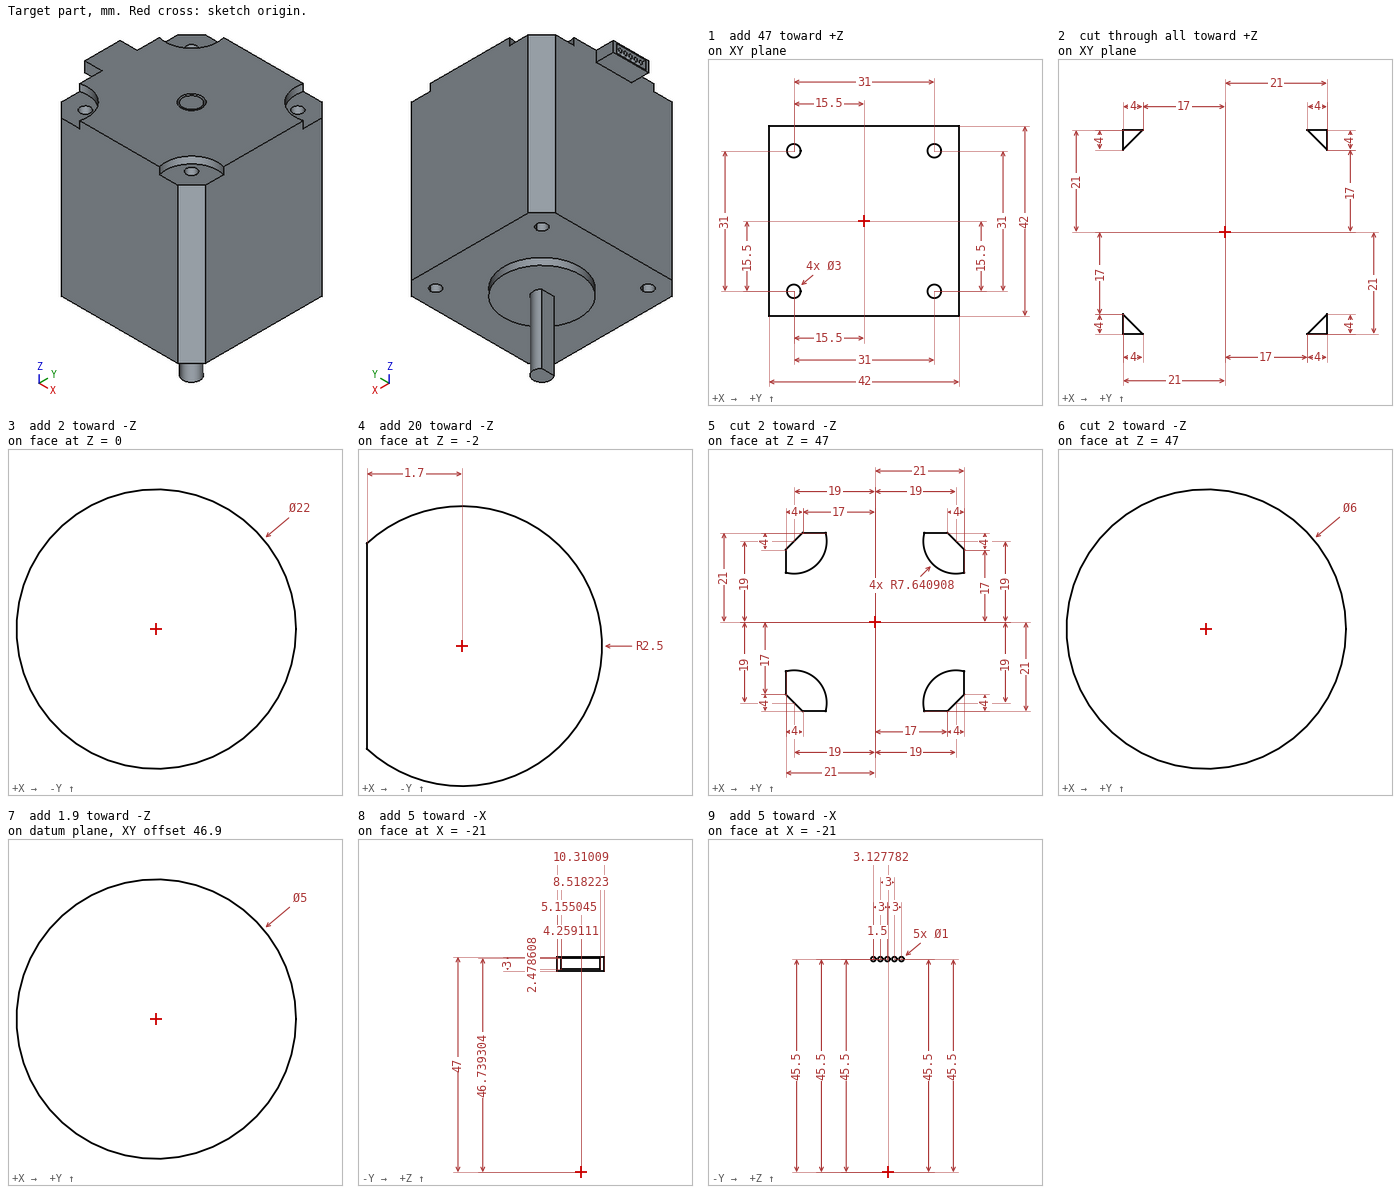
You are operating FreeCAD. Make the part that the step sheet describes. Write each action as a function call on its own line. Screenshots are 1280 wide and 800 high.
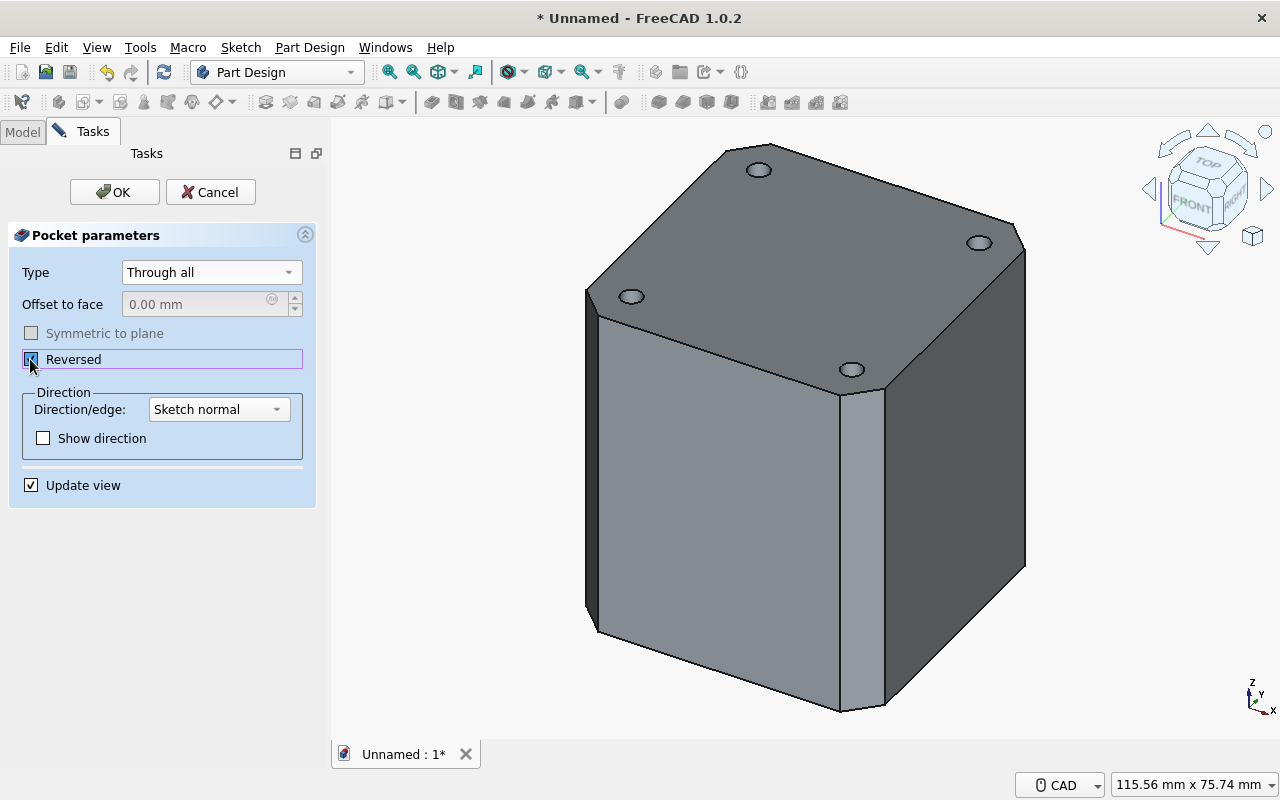
click(115, 192)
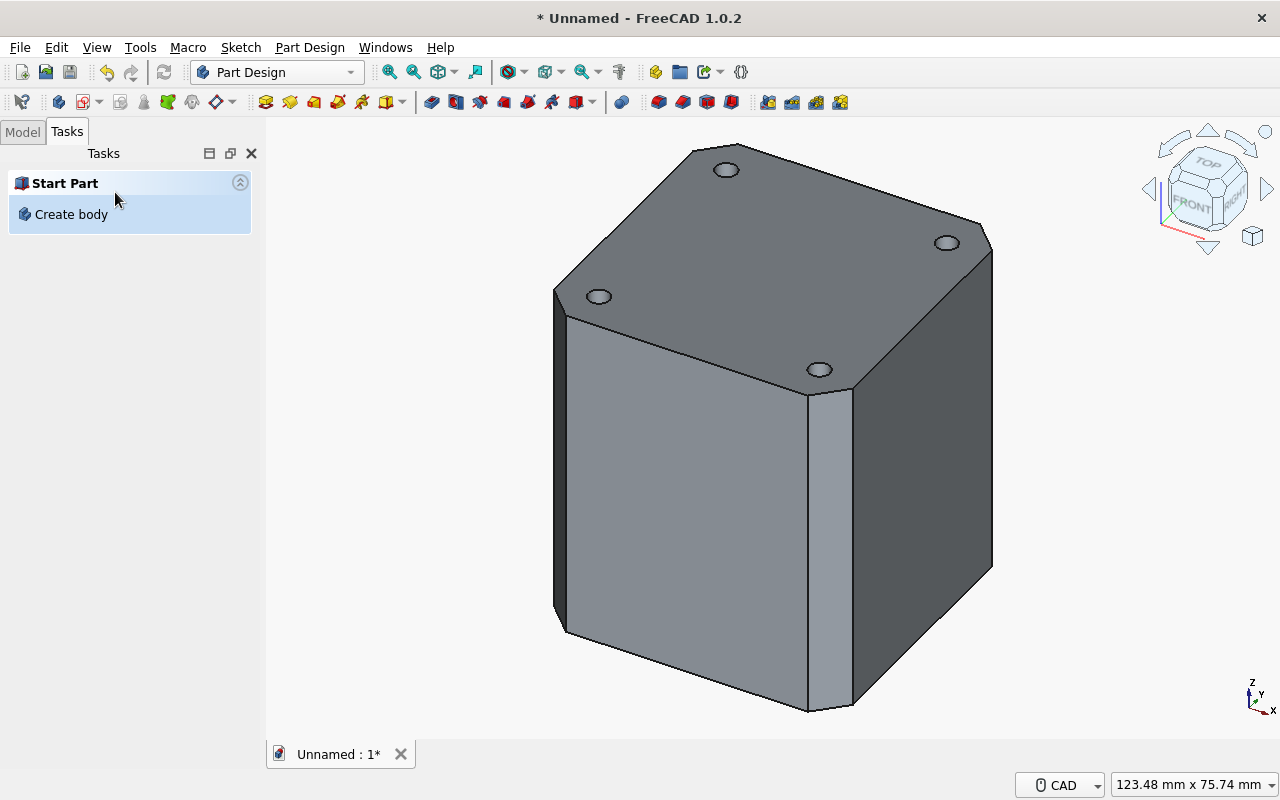
key(5)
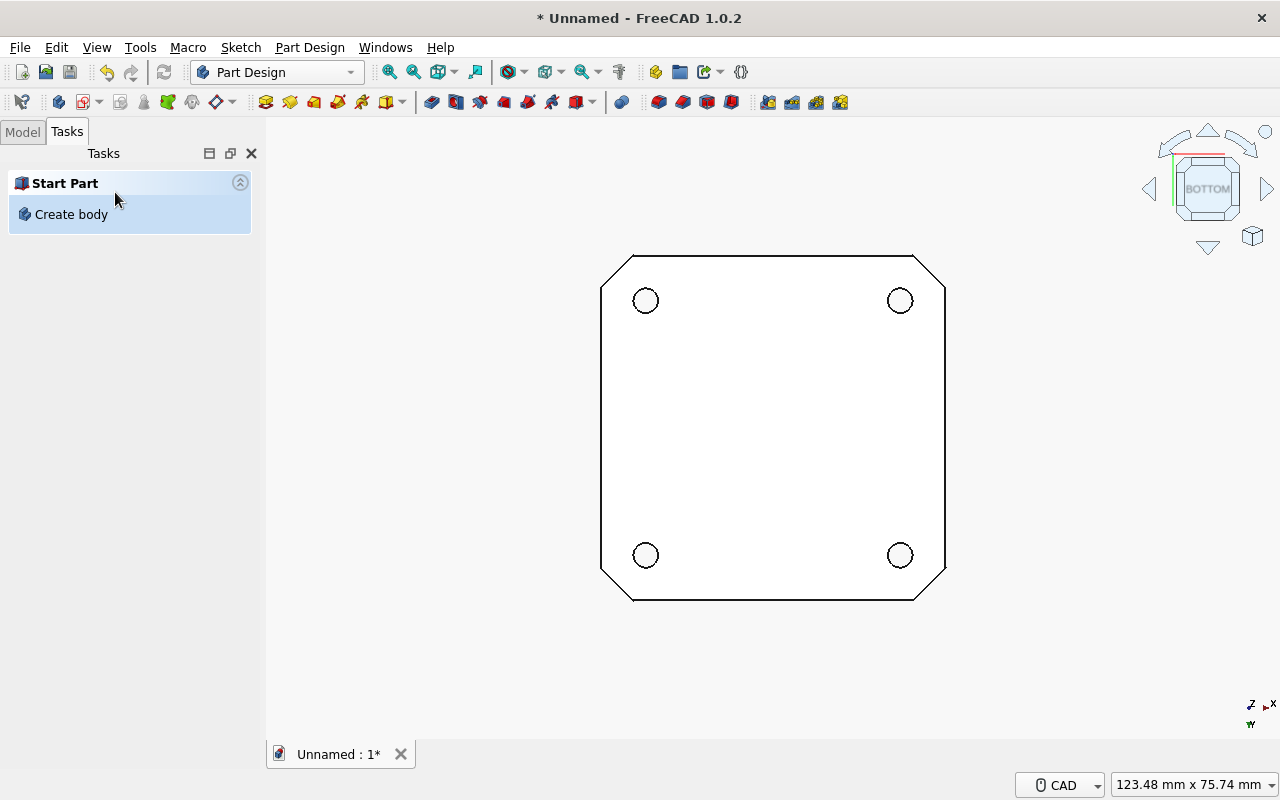
click(773, 427)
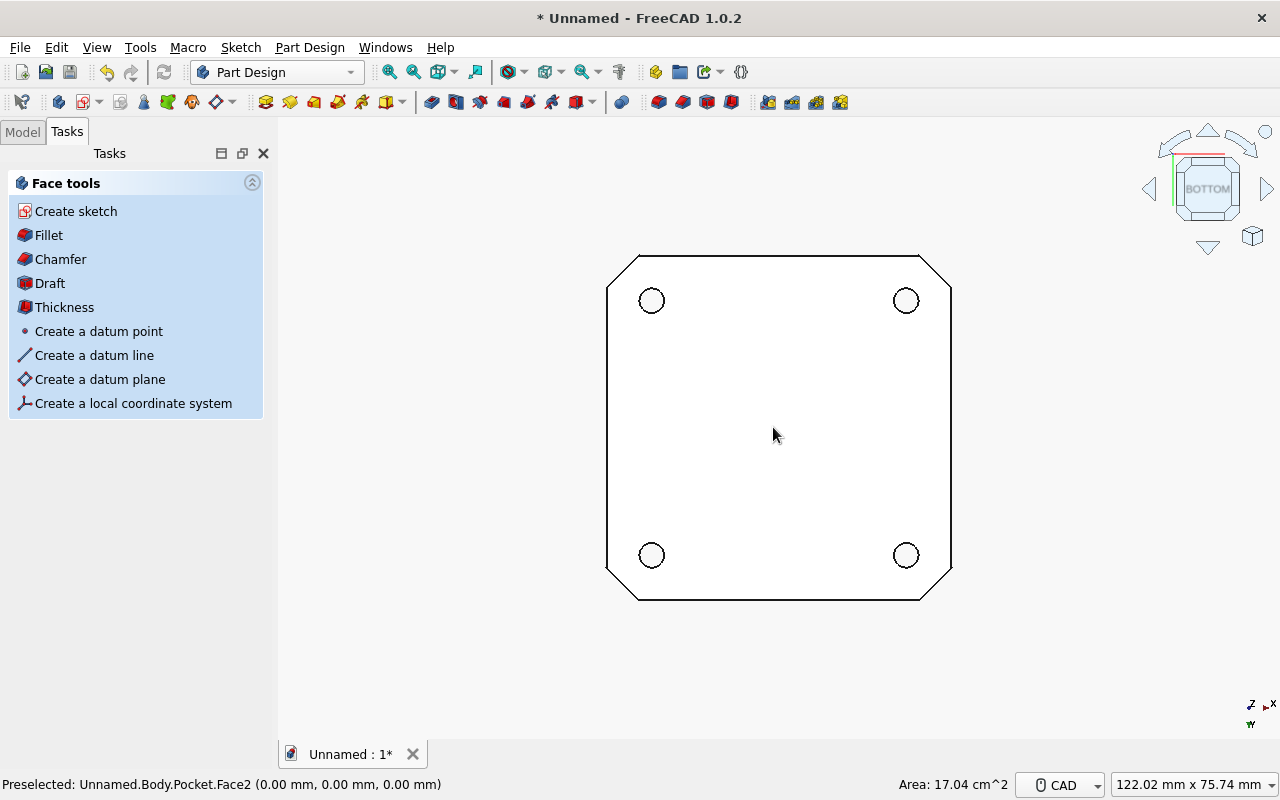
click(84, 102)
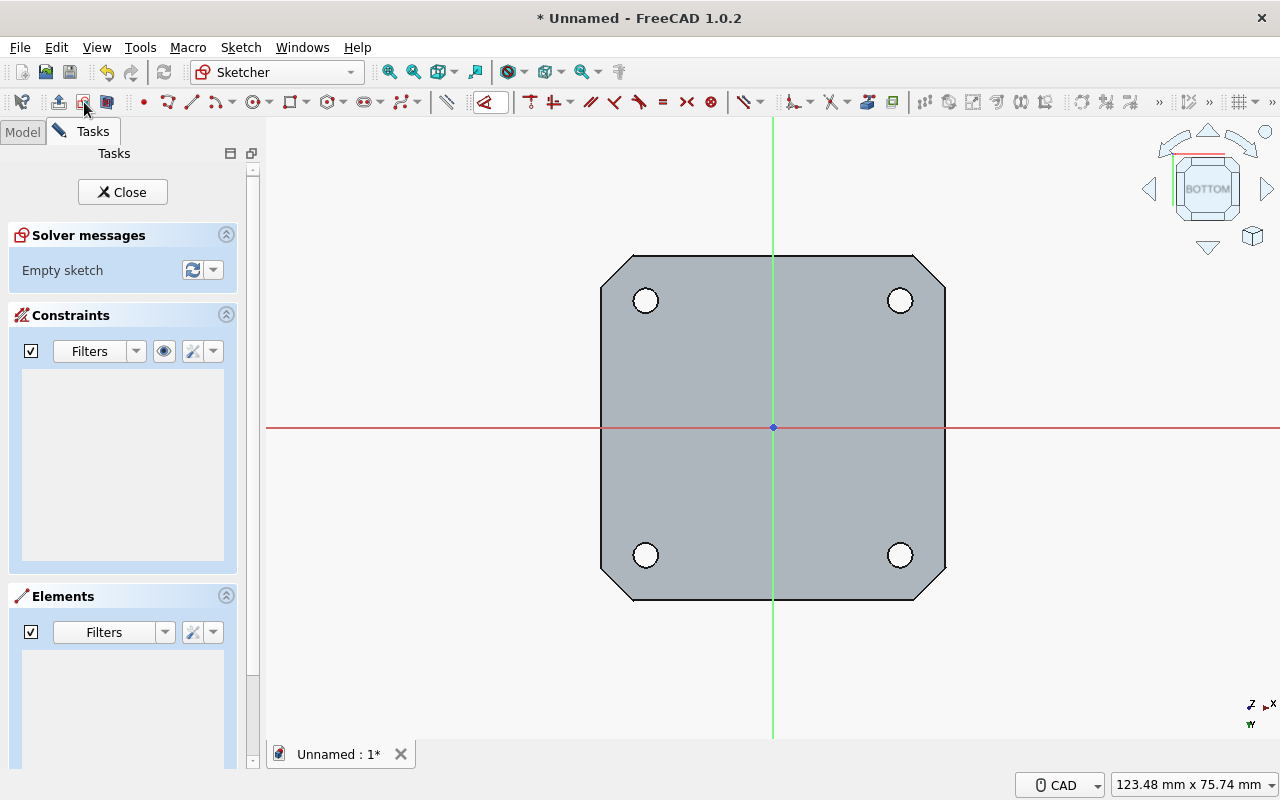
scroll(829, 428, up, 4)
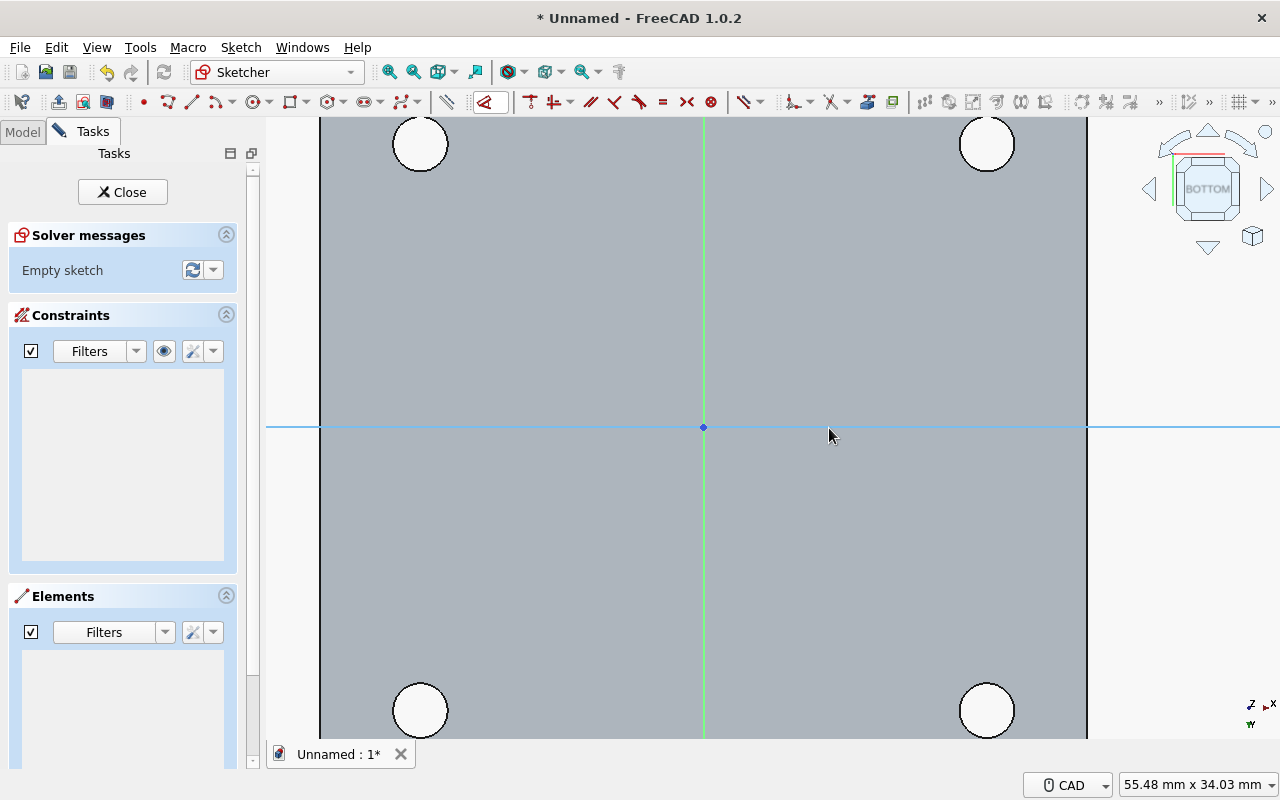
click(254, 102)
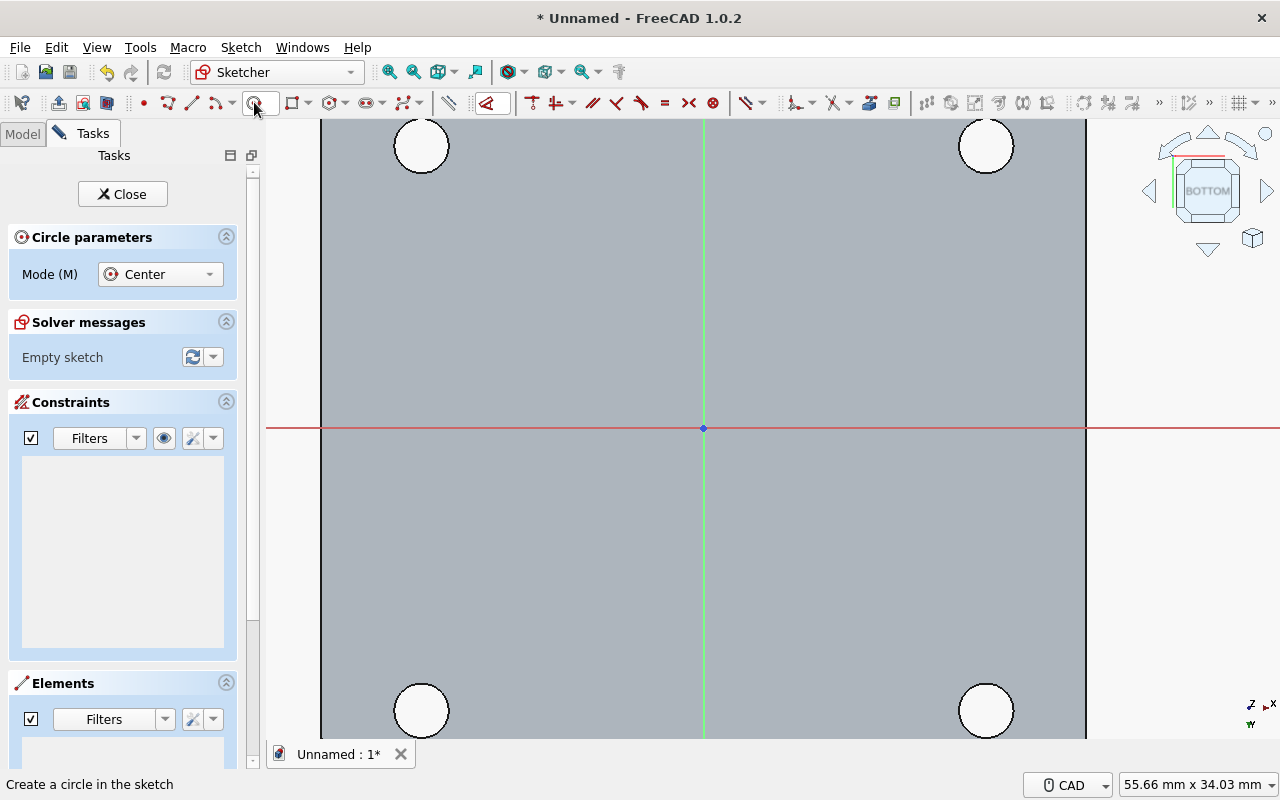
click(704, 428)
click(846, 287)
key(Escape)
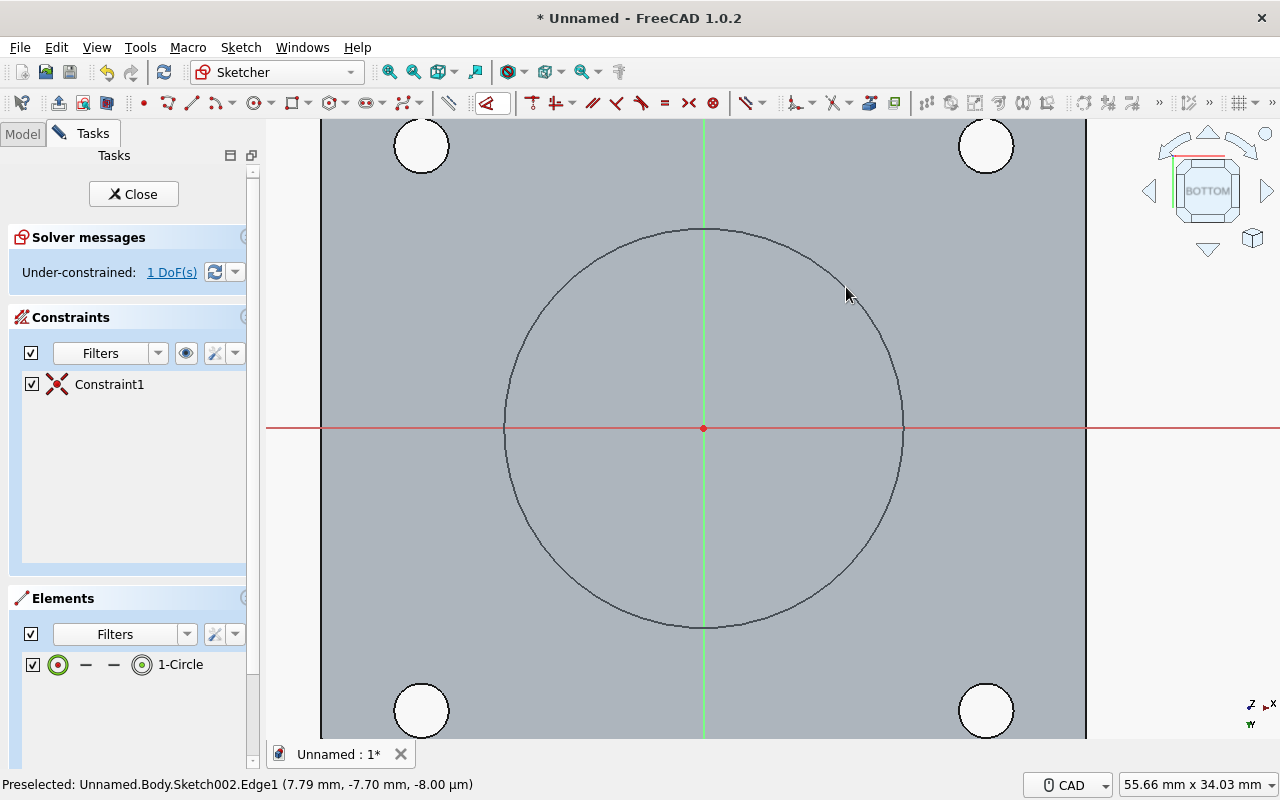
click(845, 287)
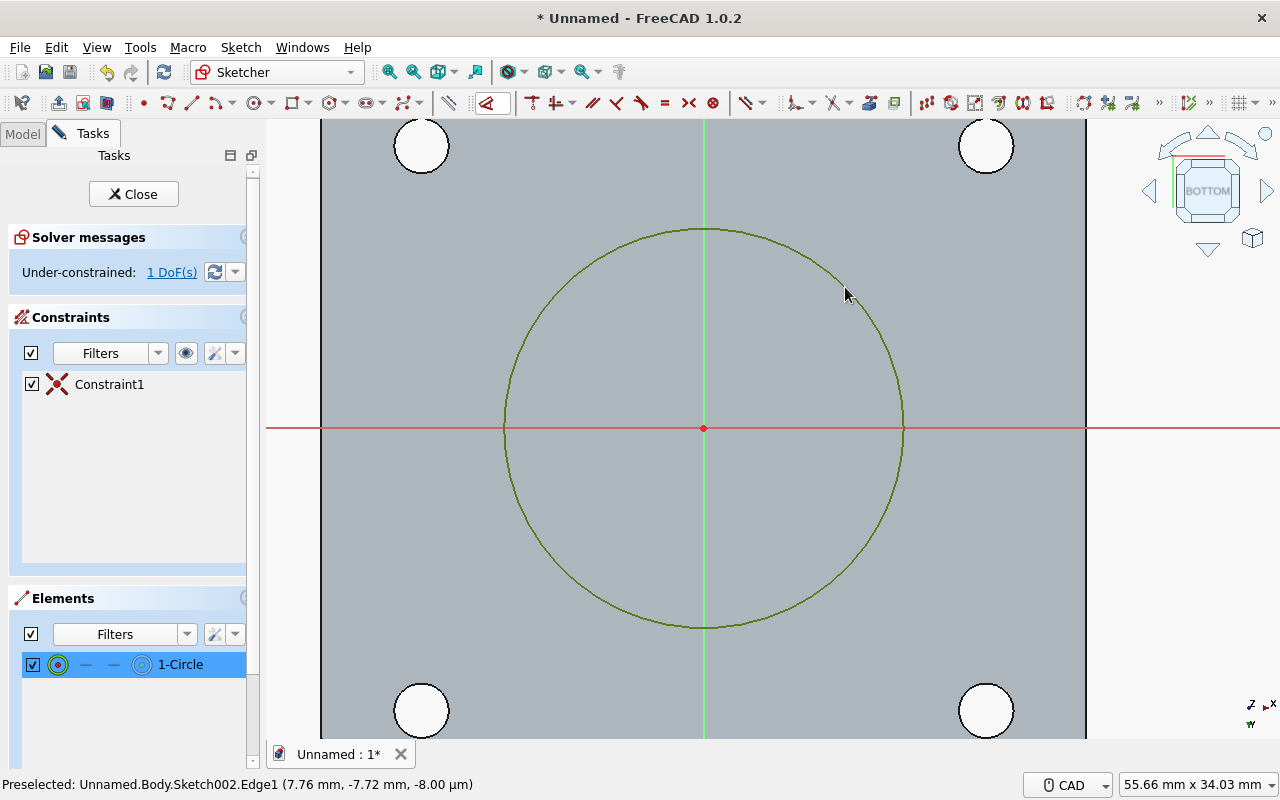
key(k)
key(o)